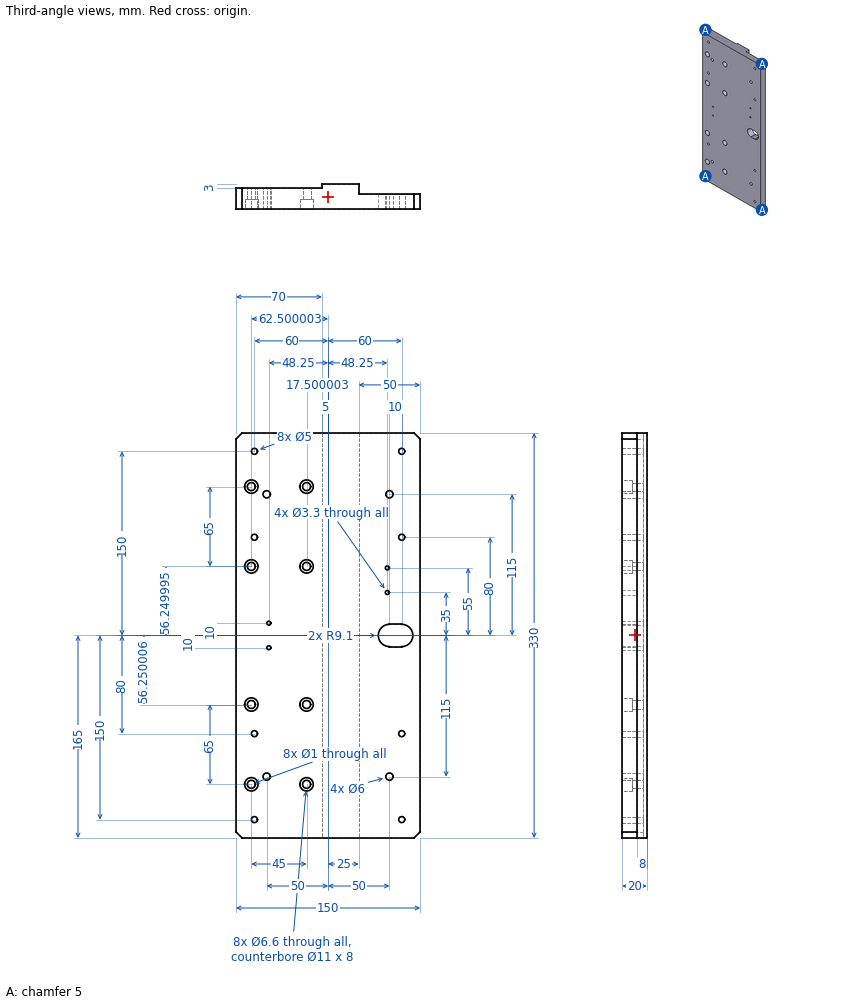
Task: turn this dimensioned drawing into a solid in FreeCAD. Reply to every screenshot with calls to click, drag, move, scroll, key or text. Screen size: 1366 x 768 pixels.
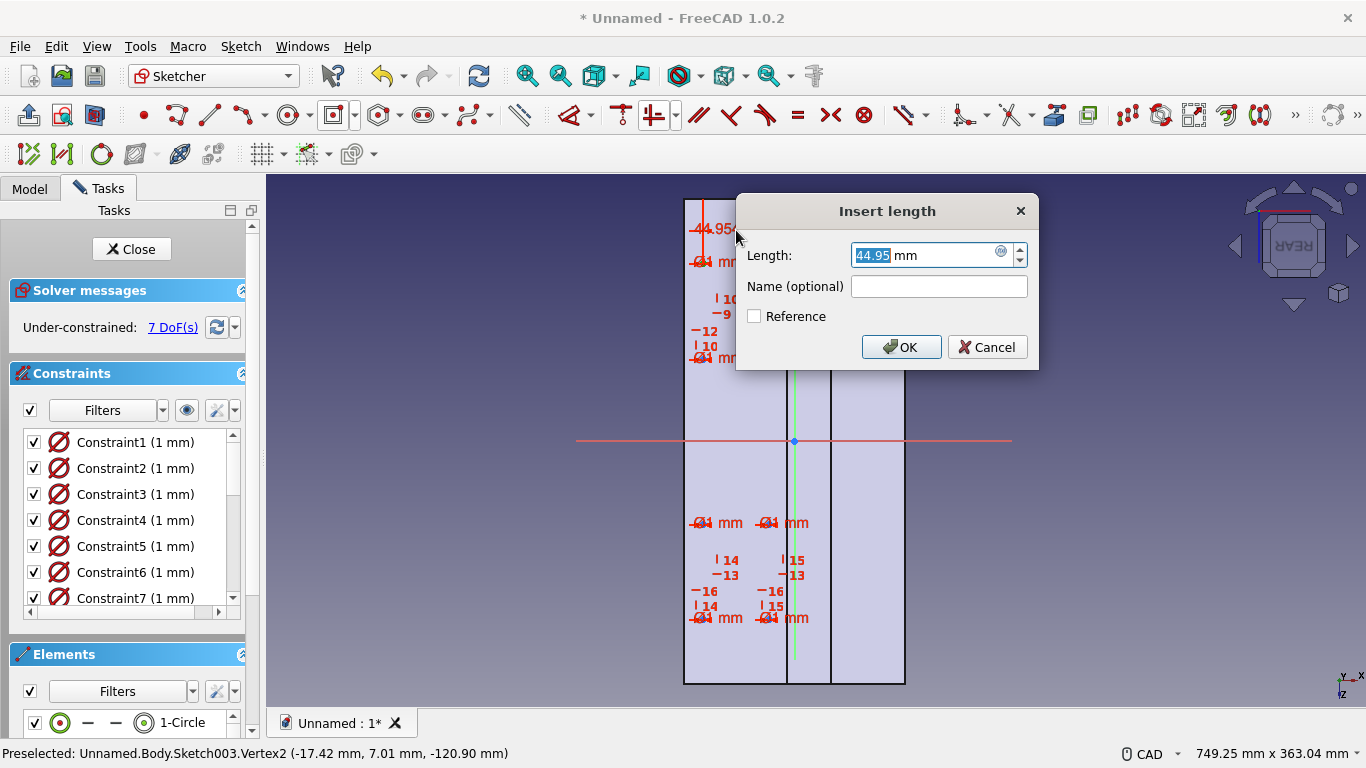
text(45)
key(Return)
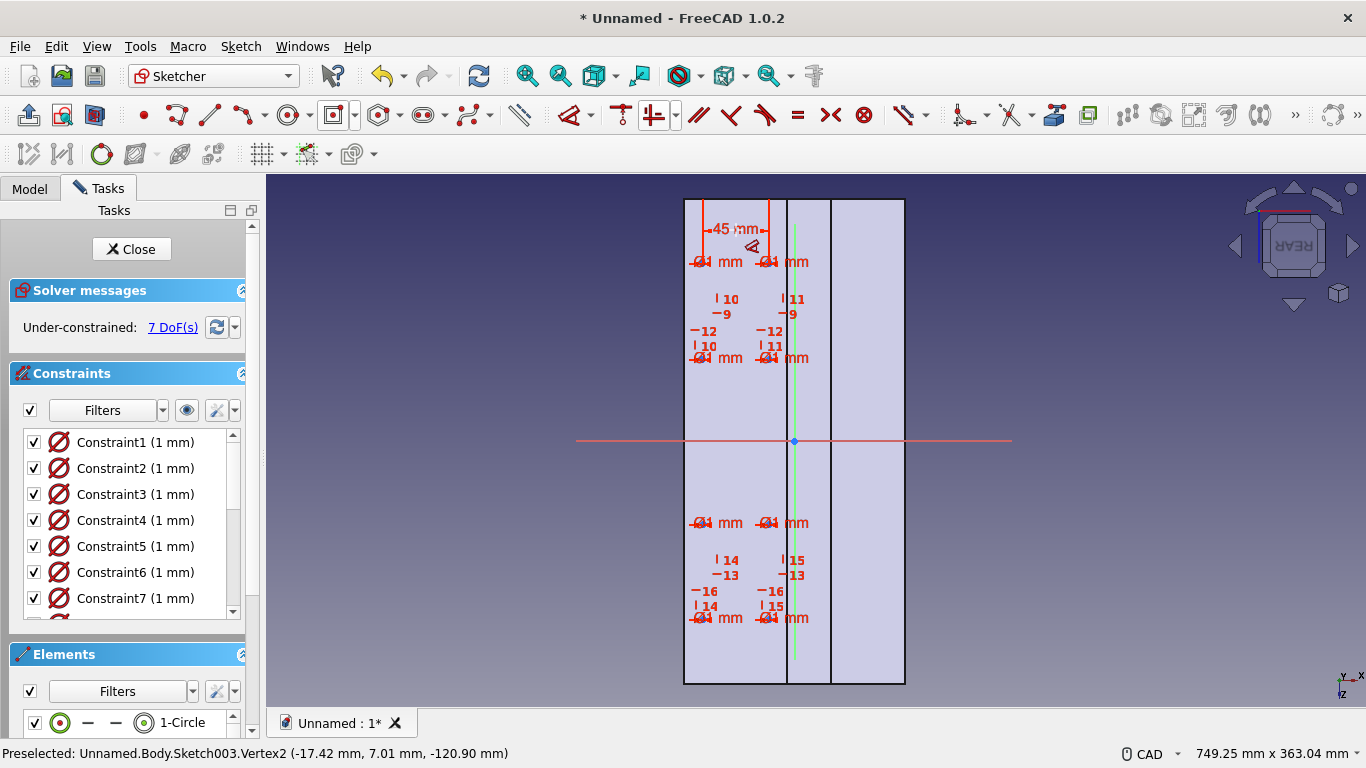
click(703, 264)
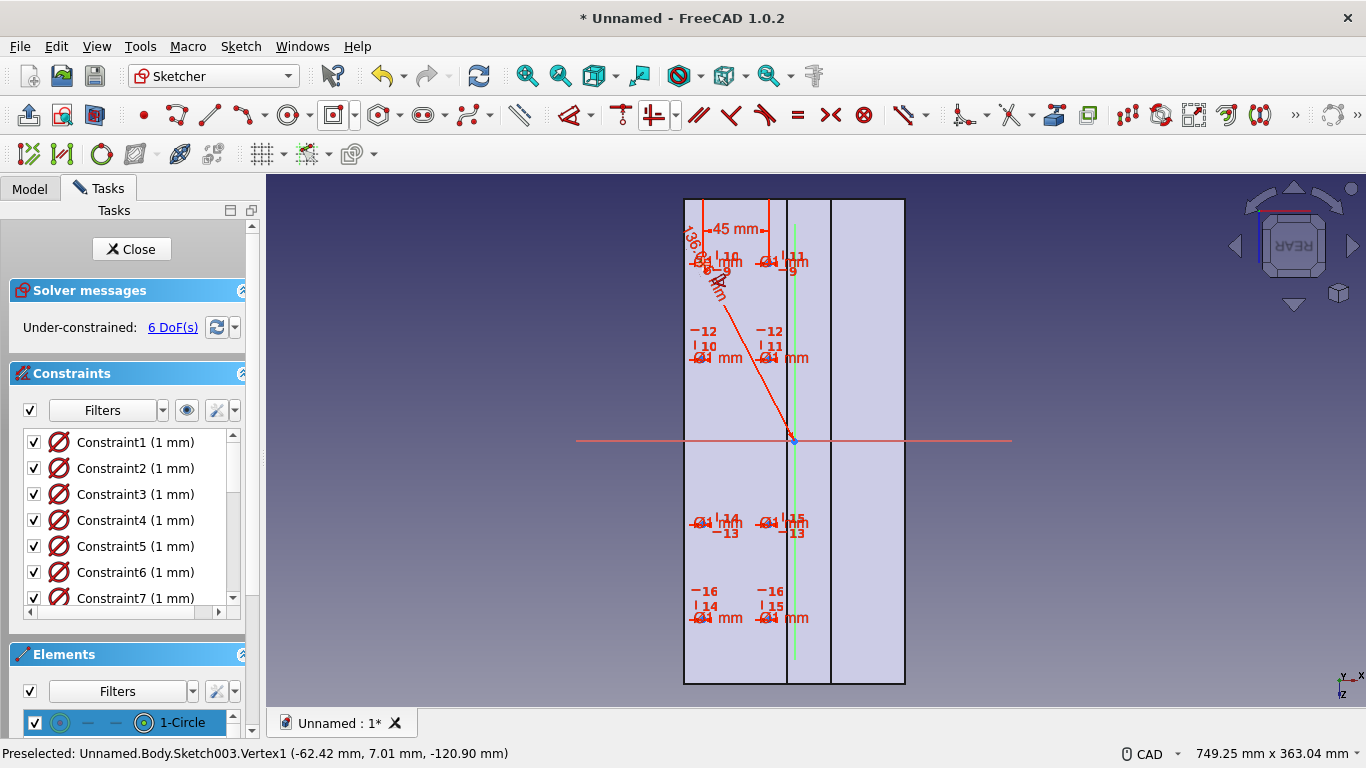
click(703, 360)
click(669, 312)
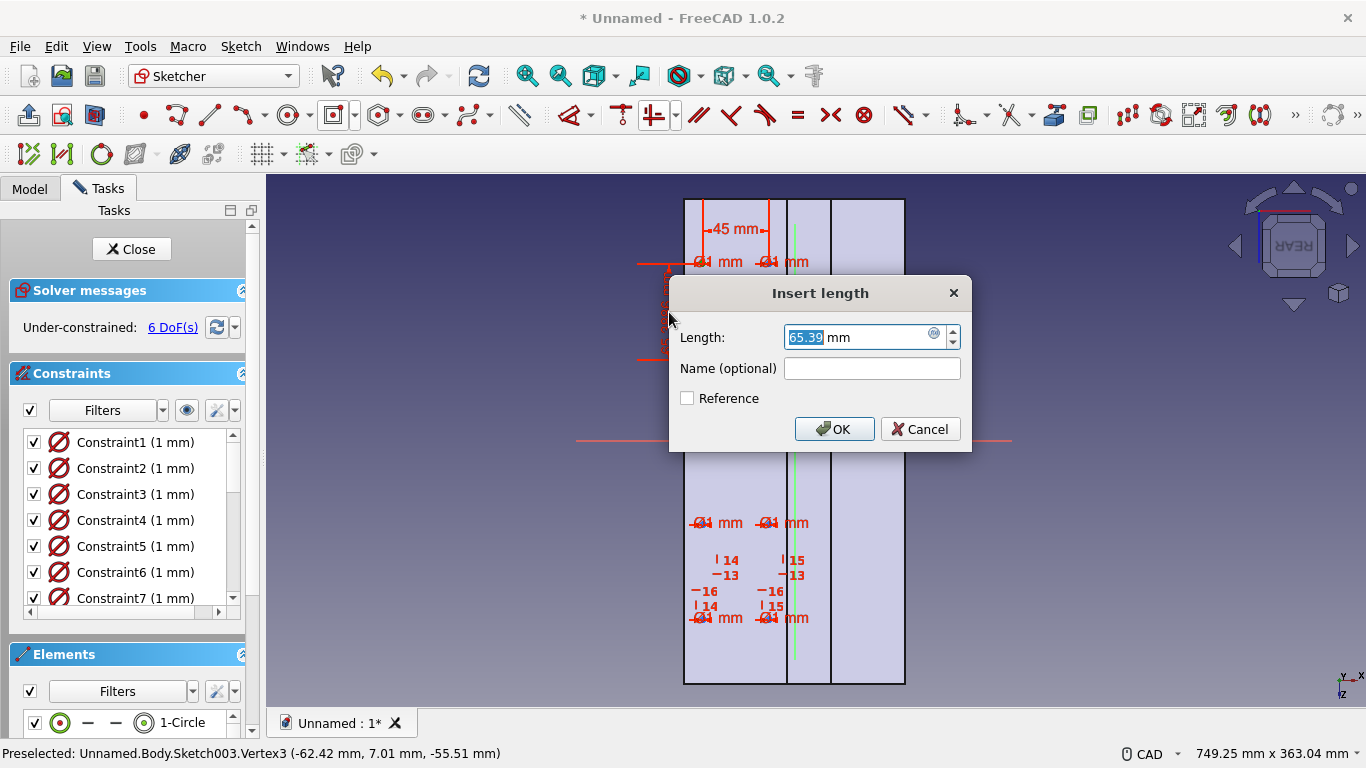
text(65)
key(Return)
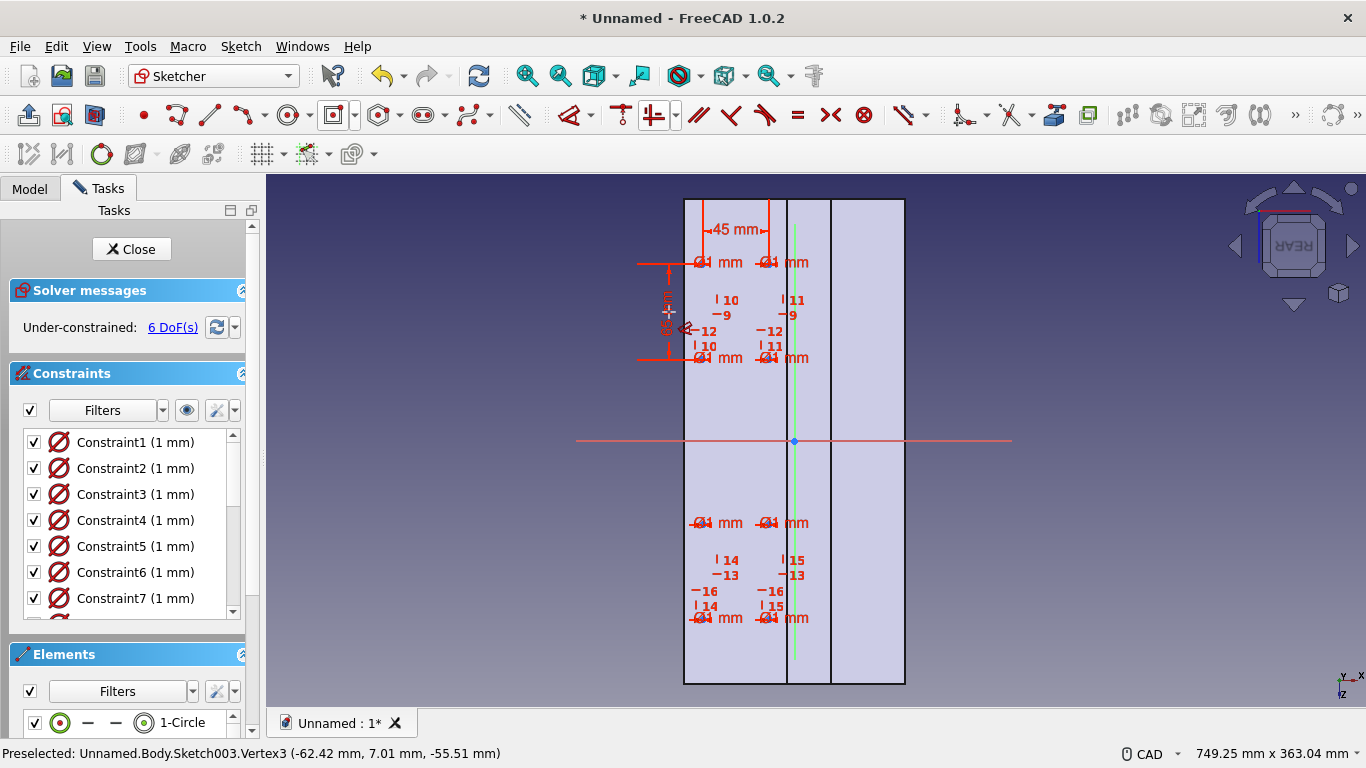
click(703, 525)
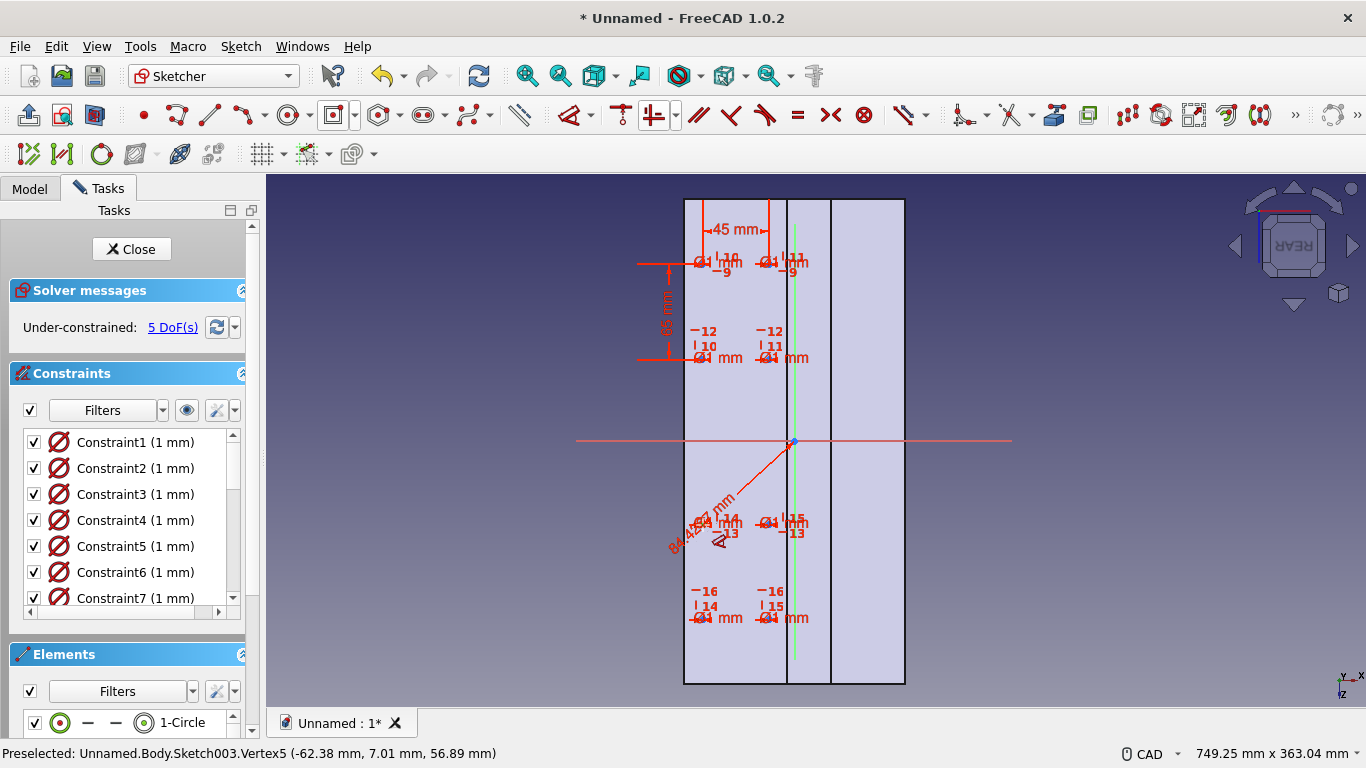
click(769, 525)
click(736, 559)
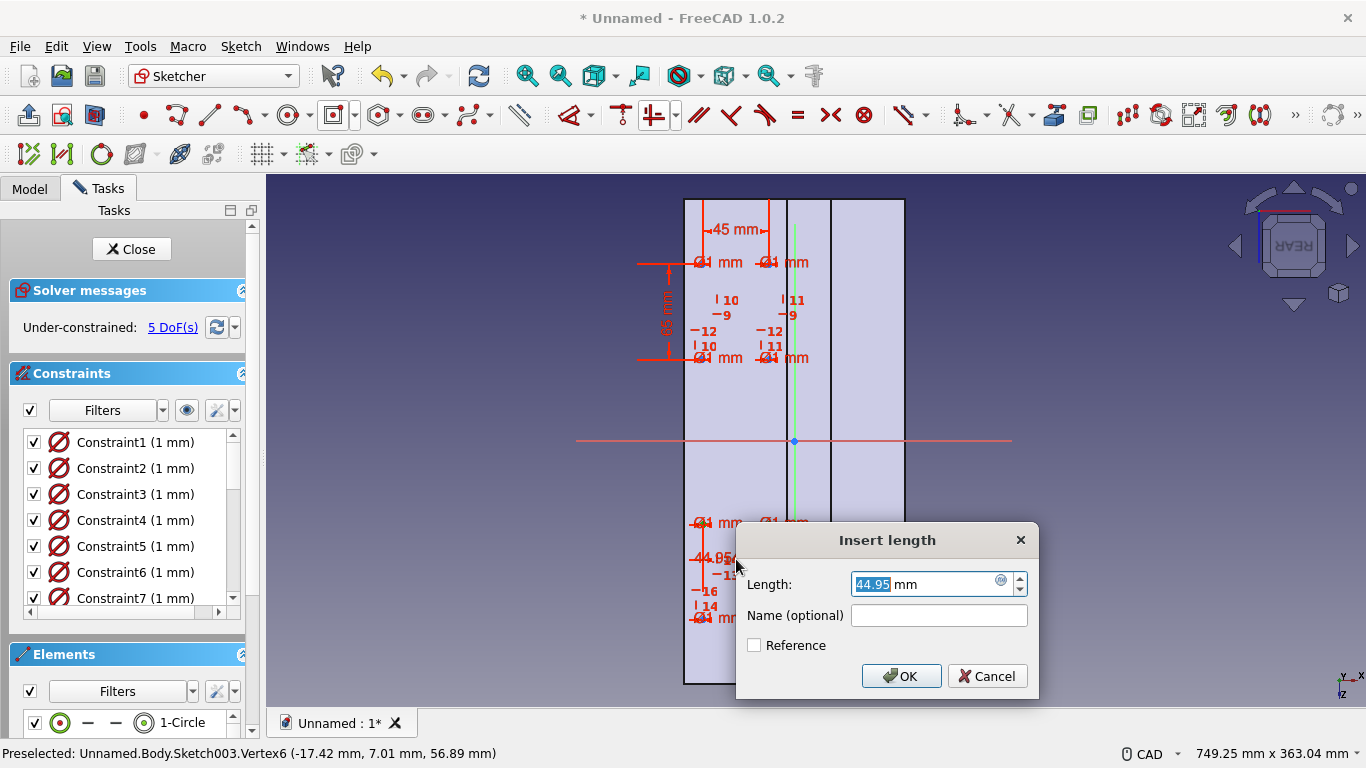
text(45)
key(Return)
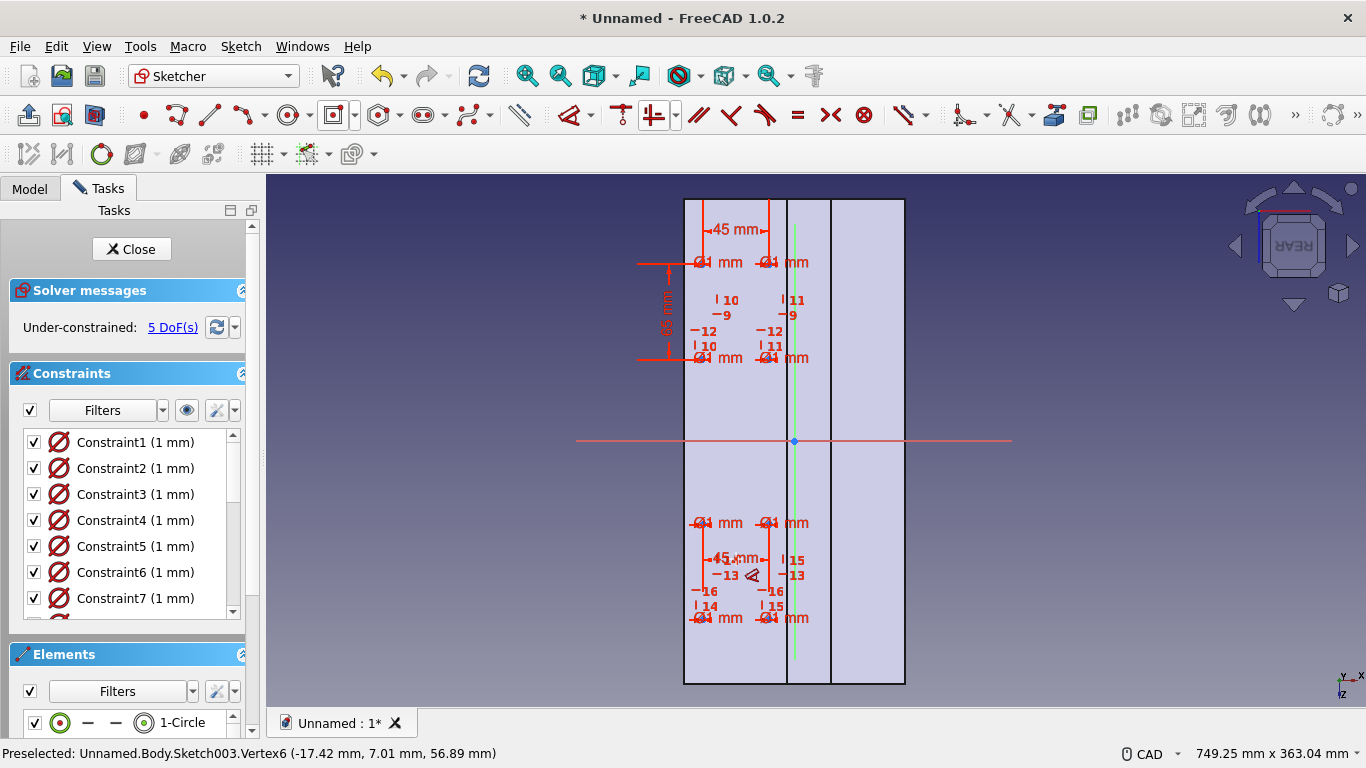
click(703, 525)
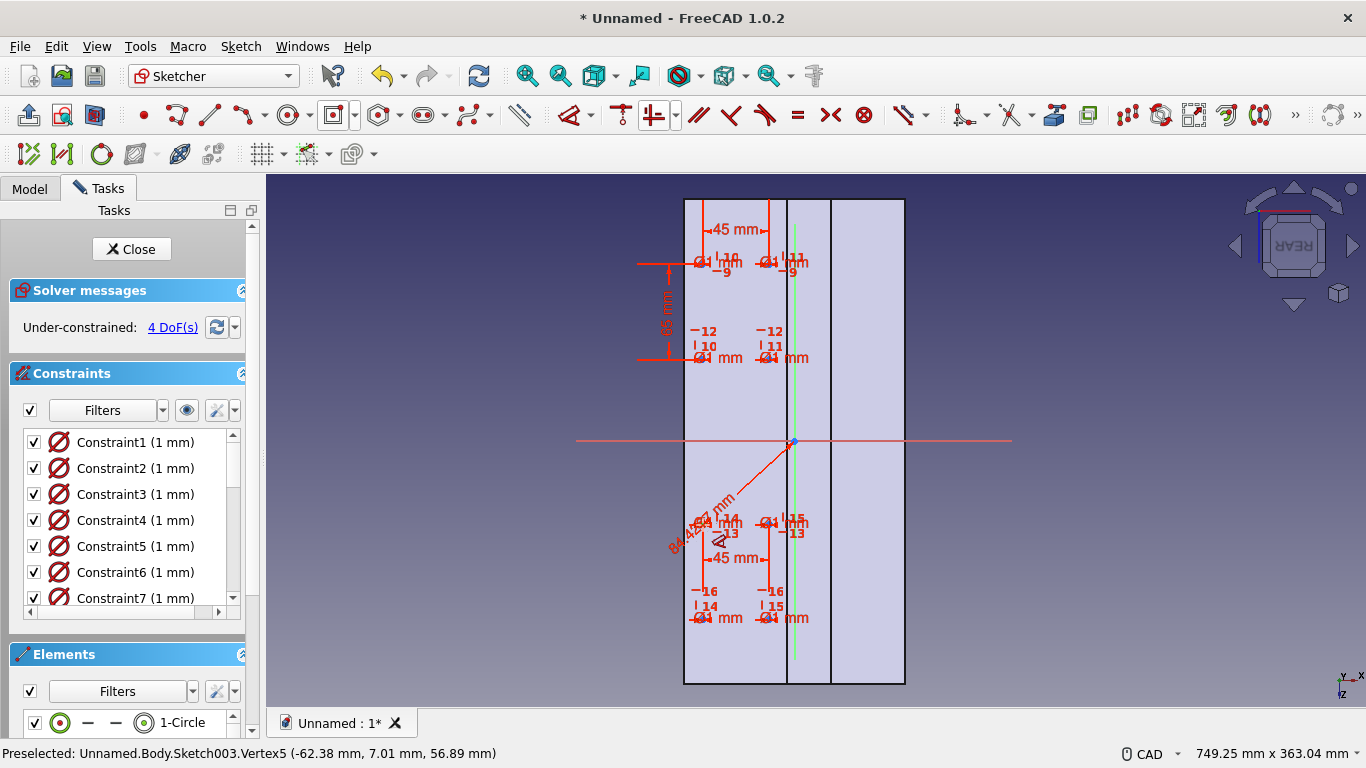
click(703, 620)
click(669, 594)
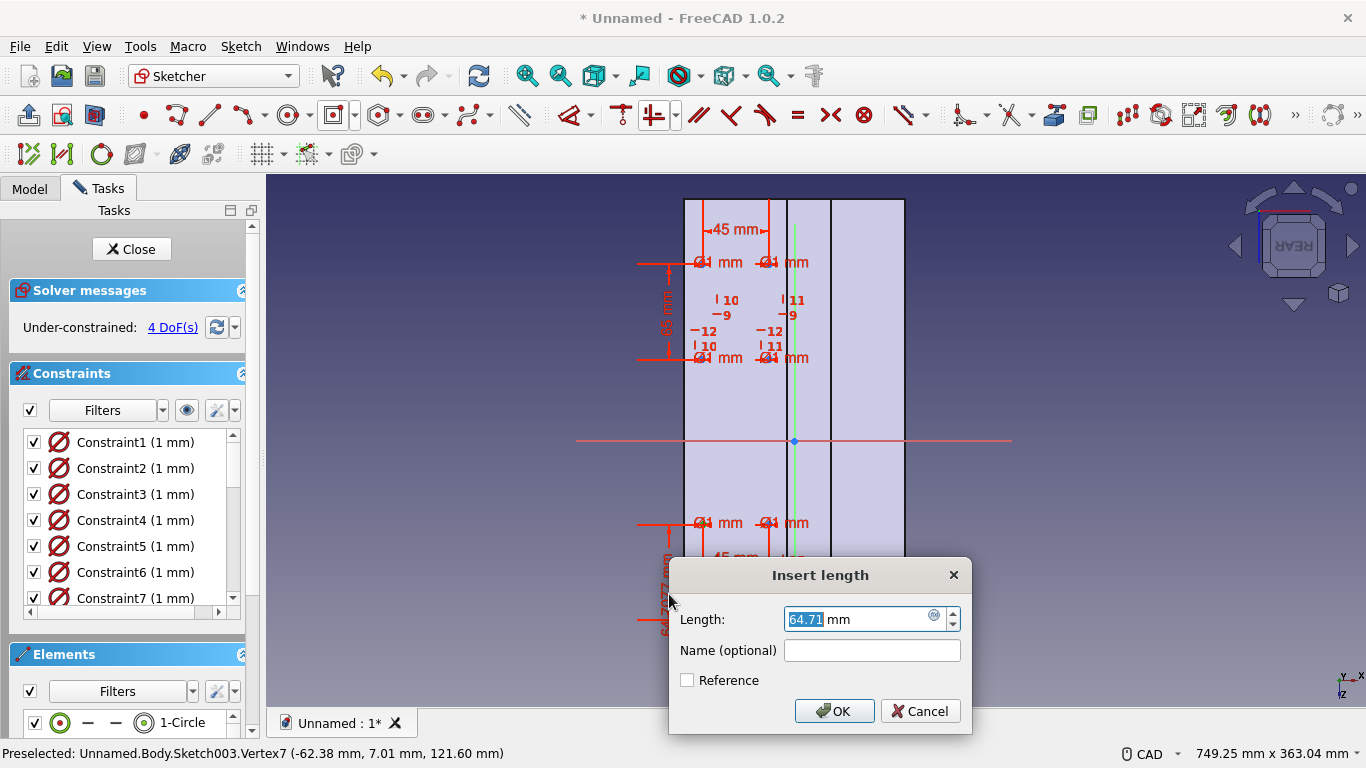
text(65)
key(Return)